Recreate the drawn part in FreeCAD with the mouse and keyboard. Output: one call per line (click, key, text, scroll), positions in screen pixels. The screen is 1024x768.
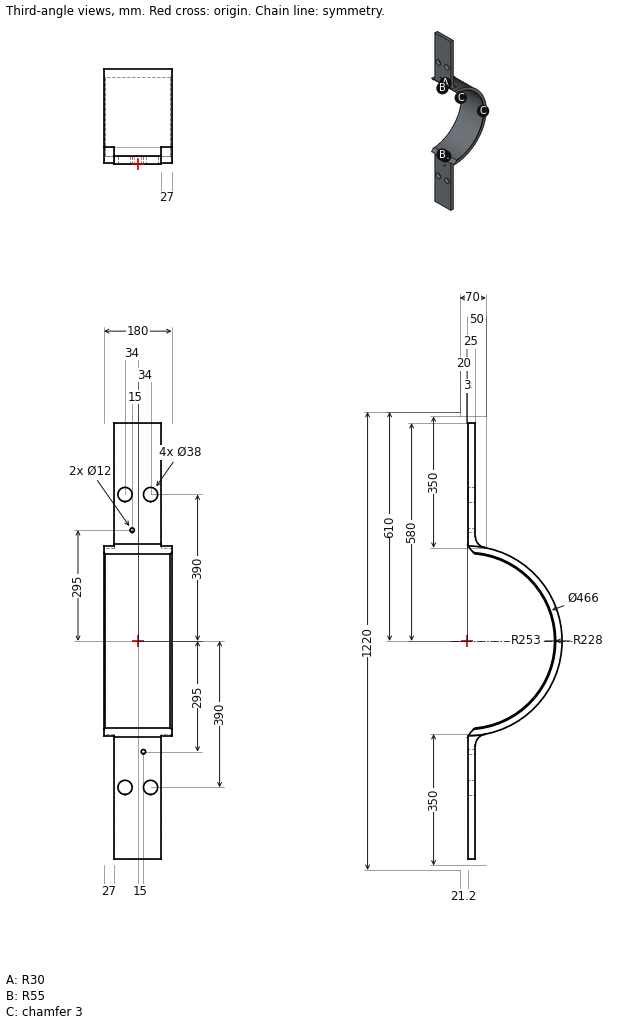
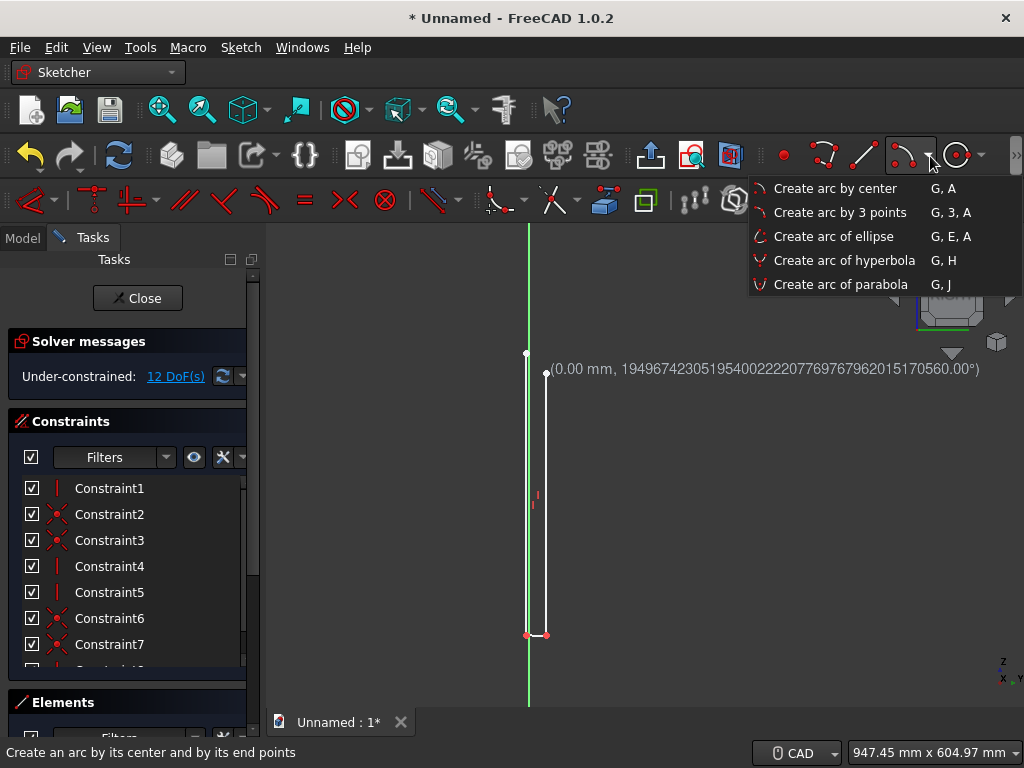
click(886, 212)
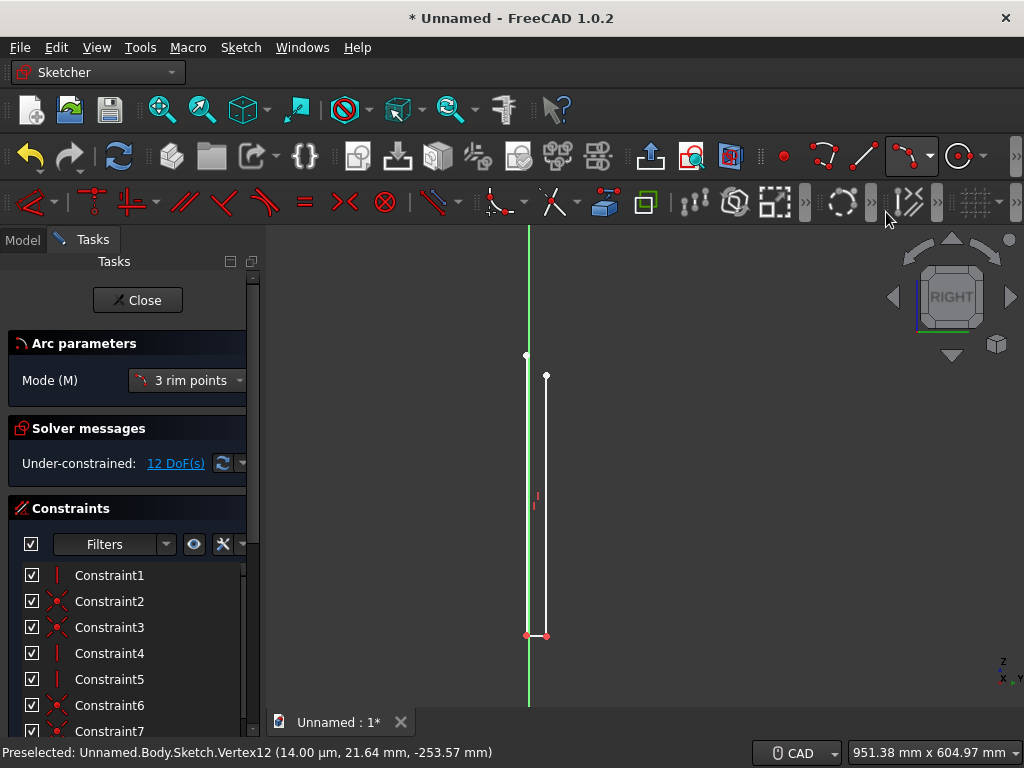
scroll(554, 592, down, 6)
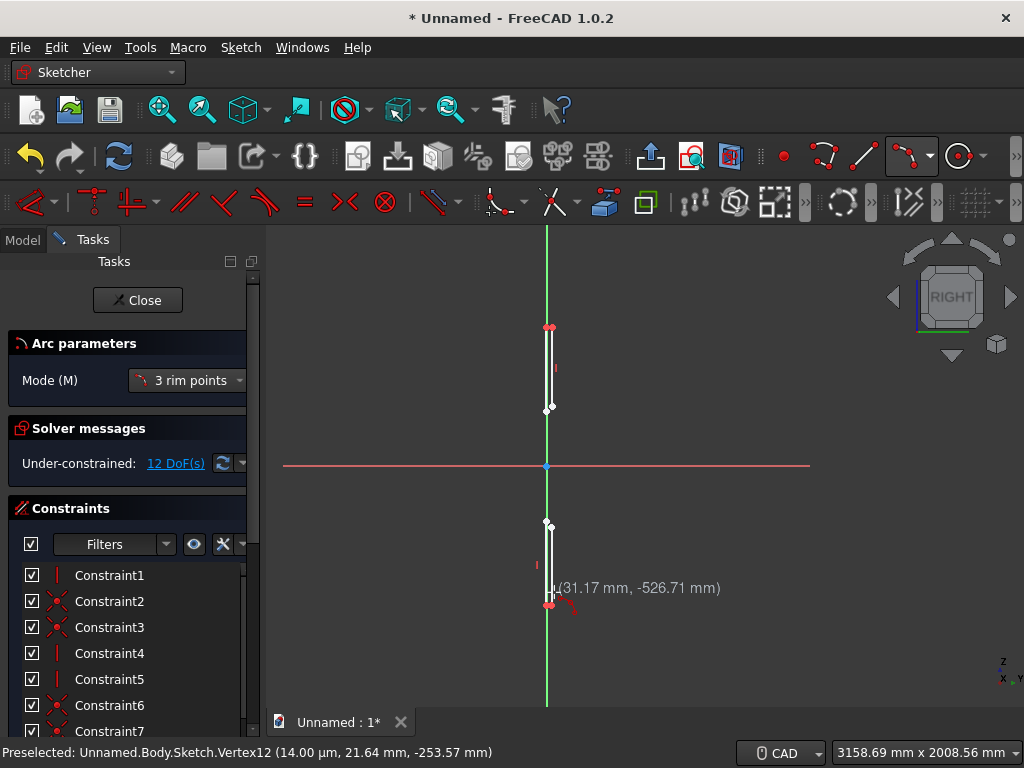
scroll(546, 412, up, 16)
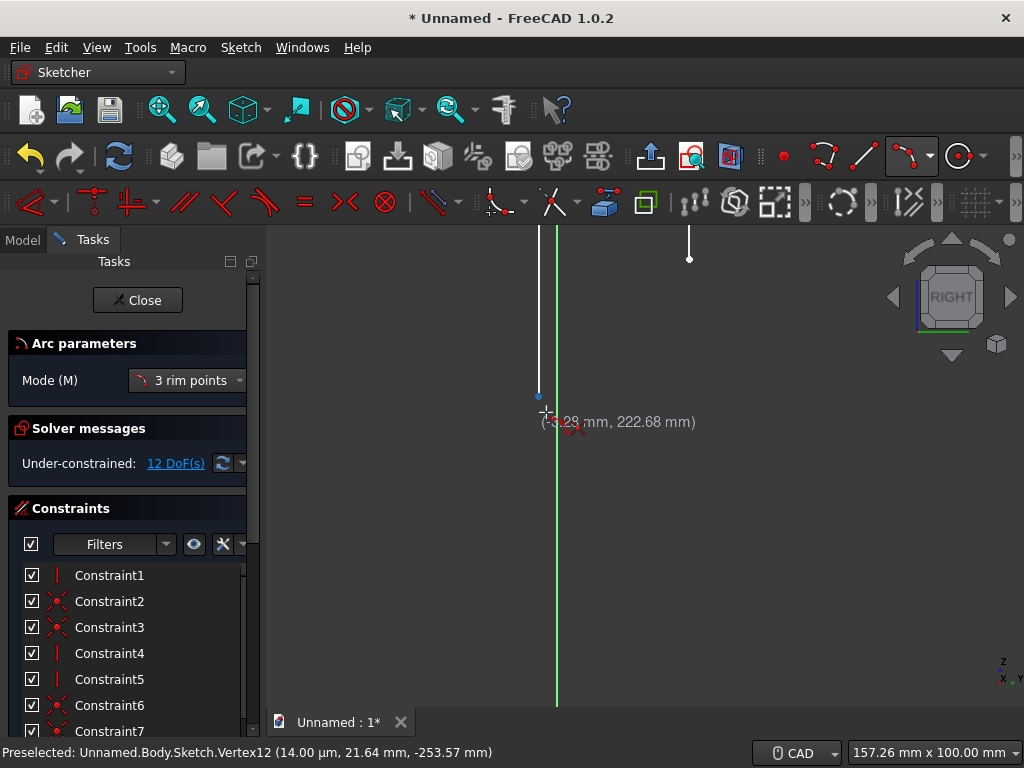
click(539, 397)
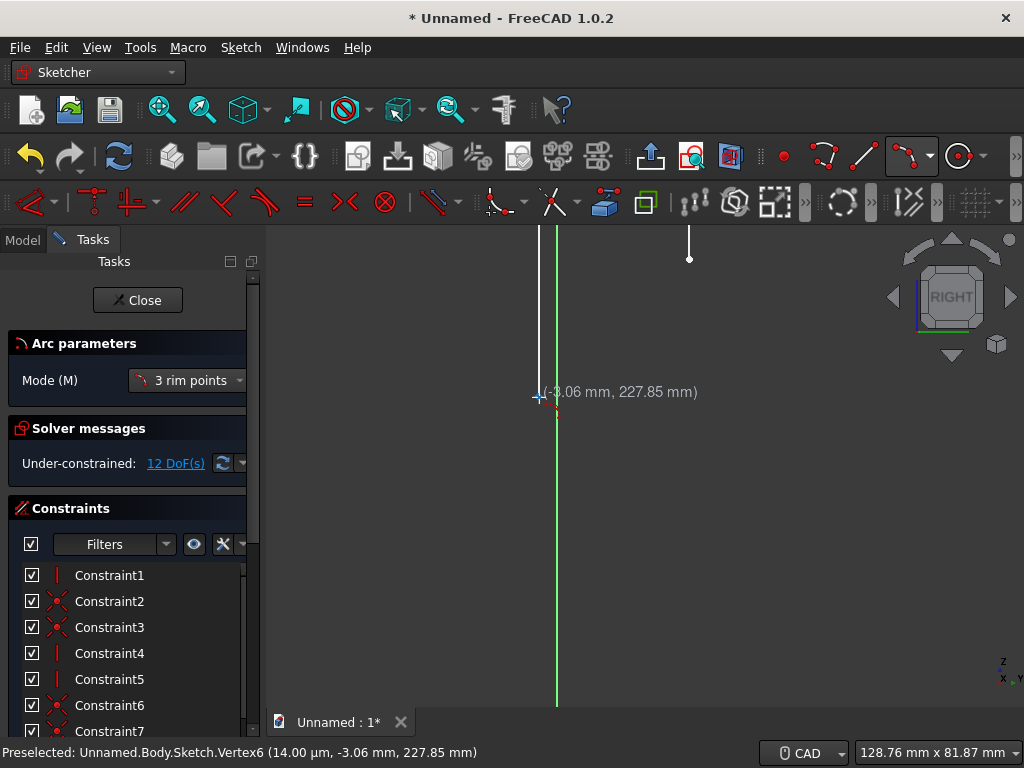
scroll(539, 399, down, 15)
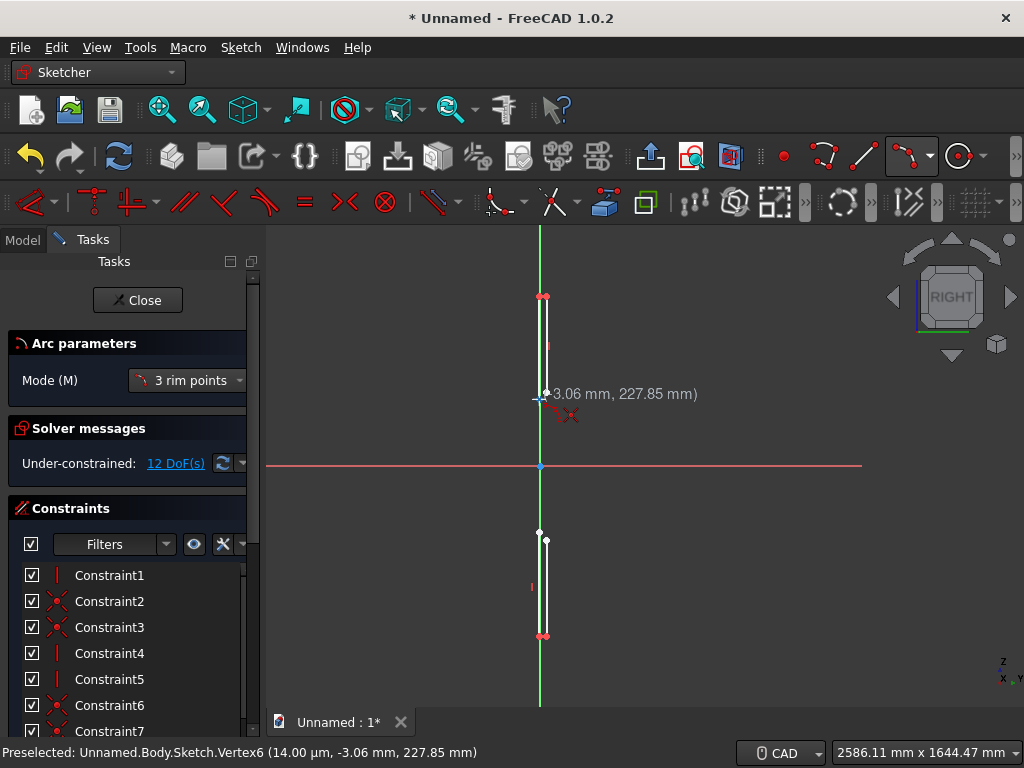
scroll(539, 533, up, 15)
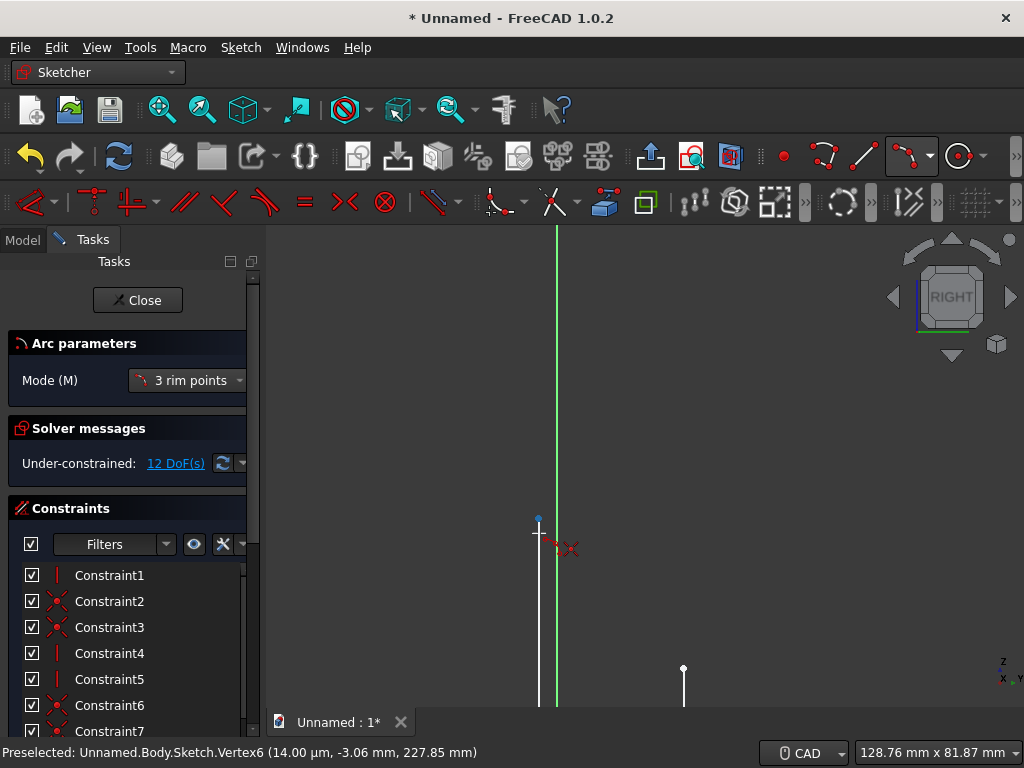
click(539, 519)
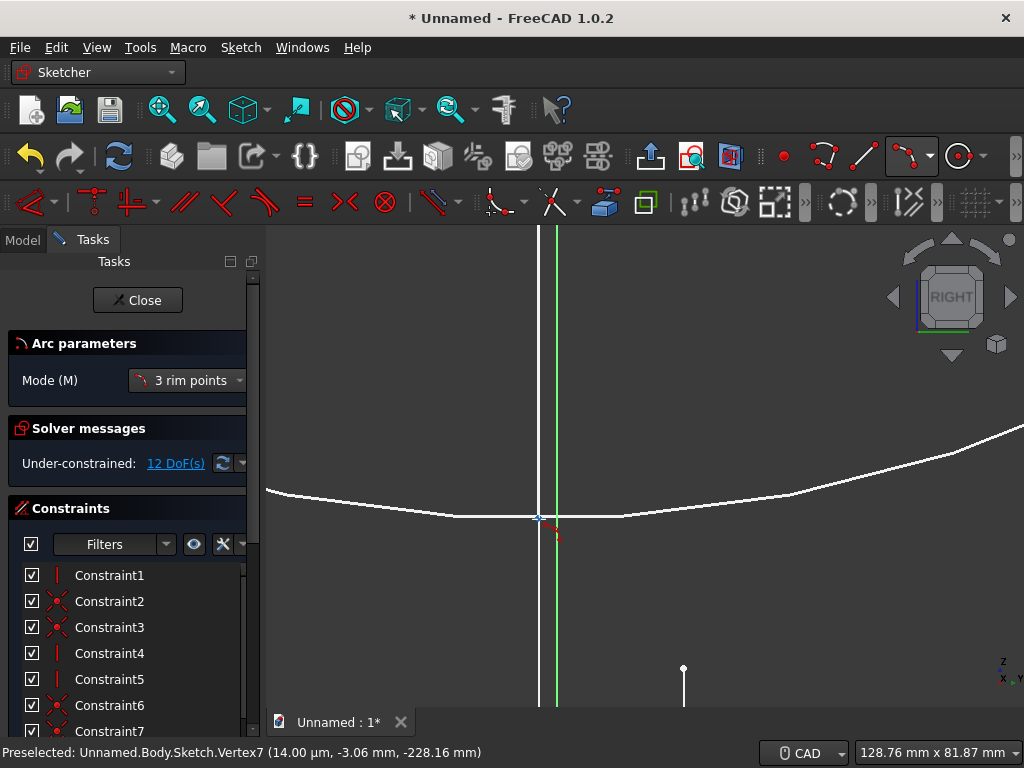
scroll(539, 534, down, 15)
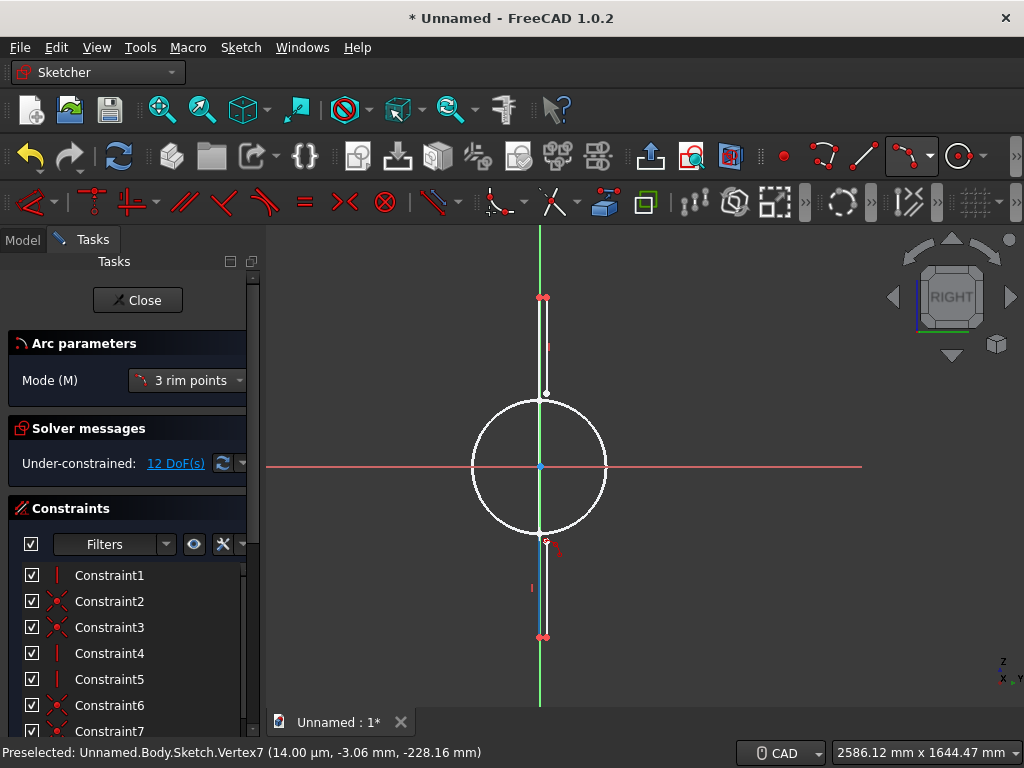
click(604, 488)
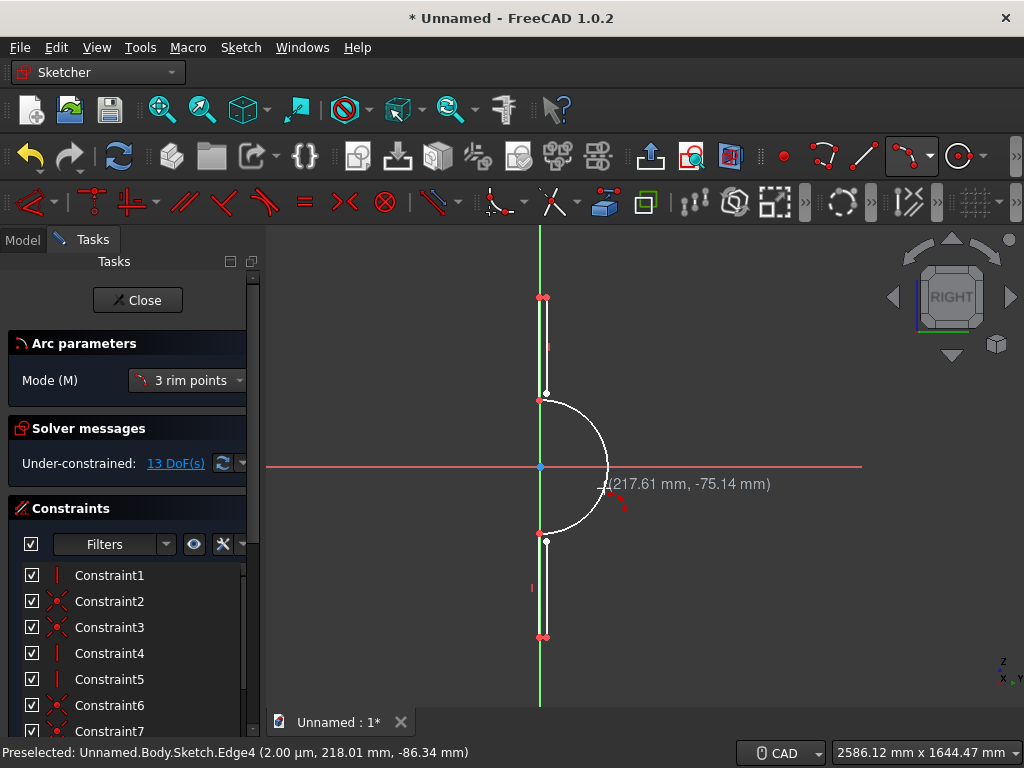
scroll(547, 541, up, 5)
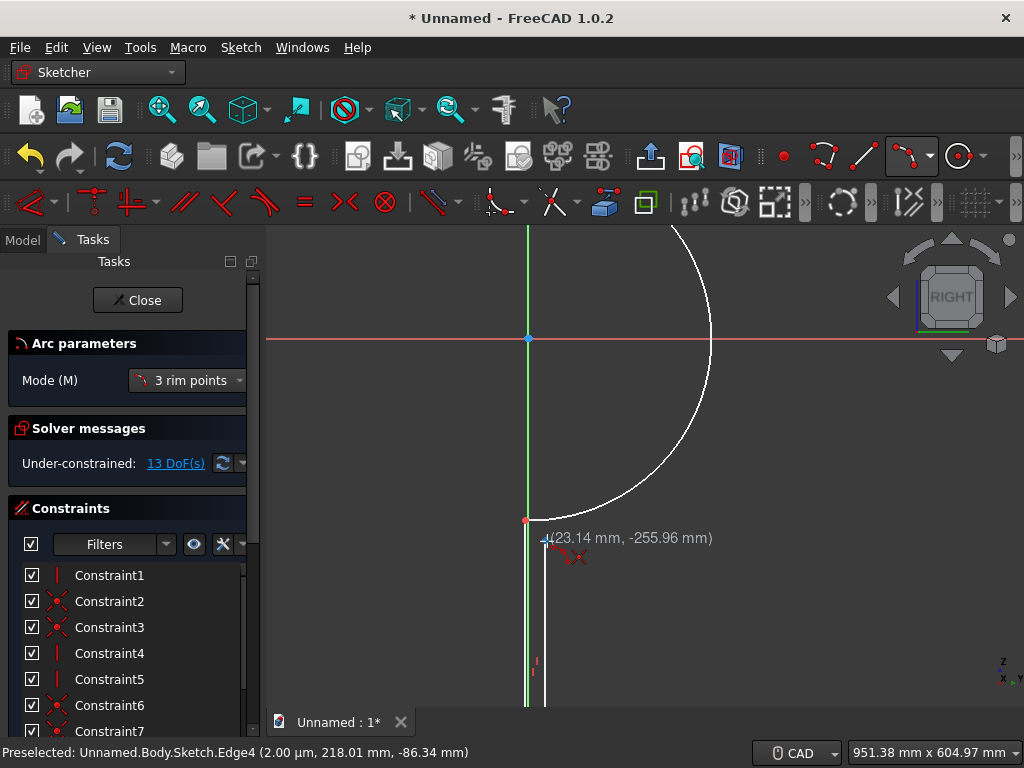
click(545, 541)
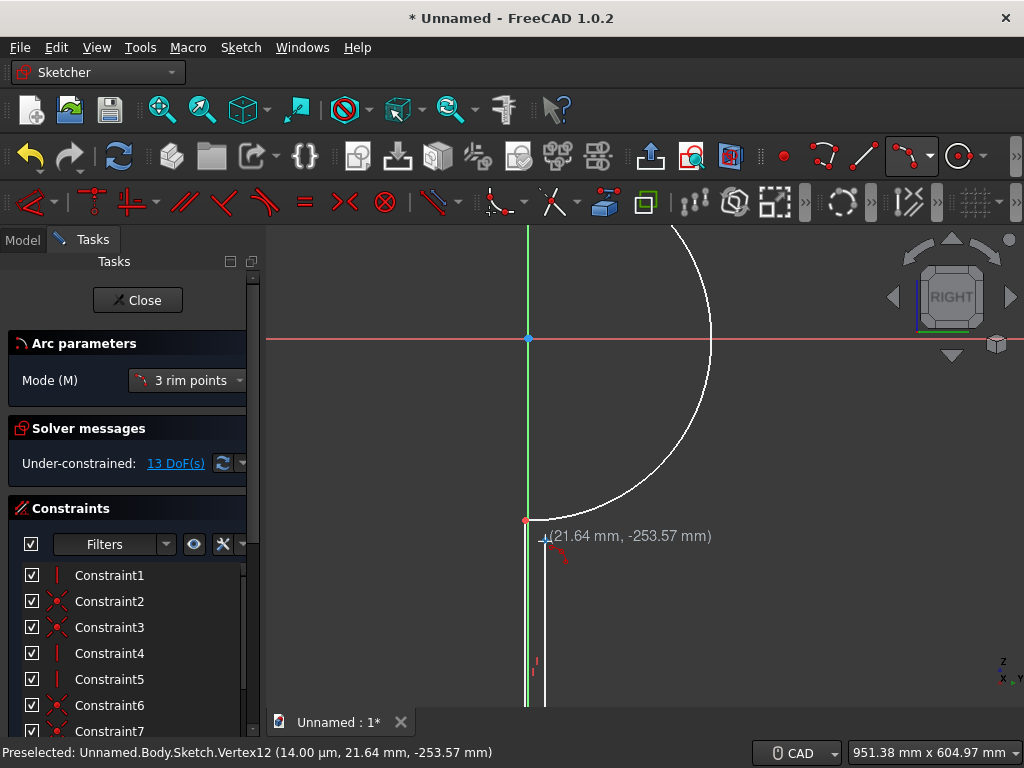
scroll(555, 521, down, 6)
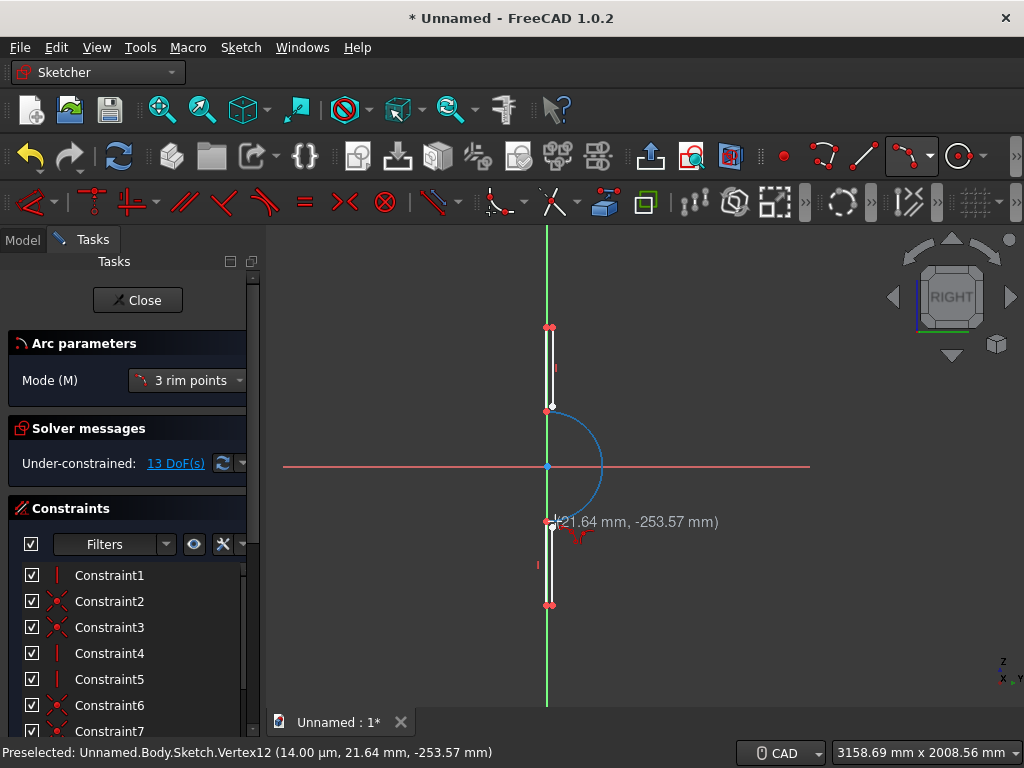
scroll(552, 406, up, 6)